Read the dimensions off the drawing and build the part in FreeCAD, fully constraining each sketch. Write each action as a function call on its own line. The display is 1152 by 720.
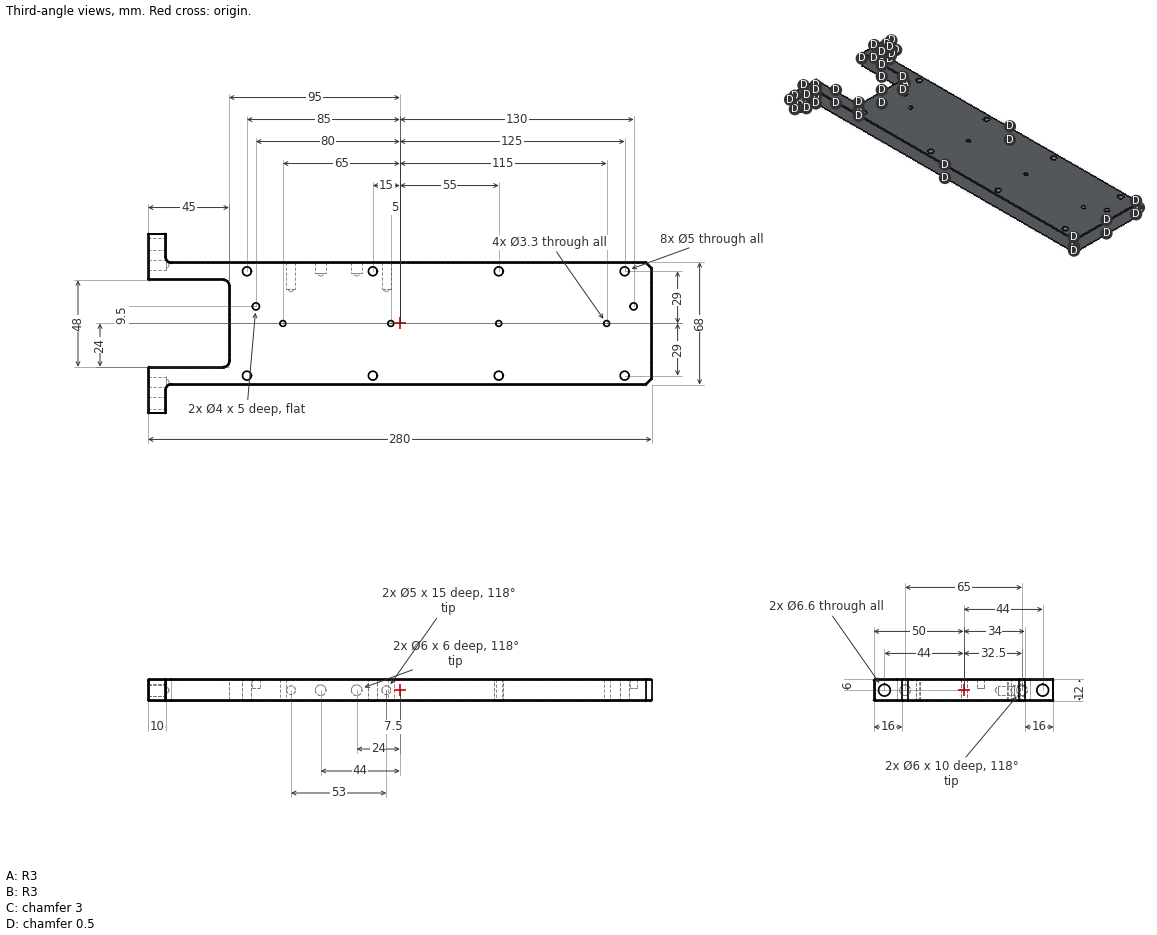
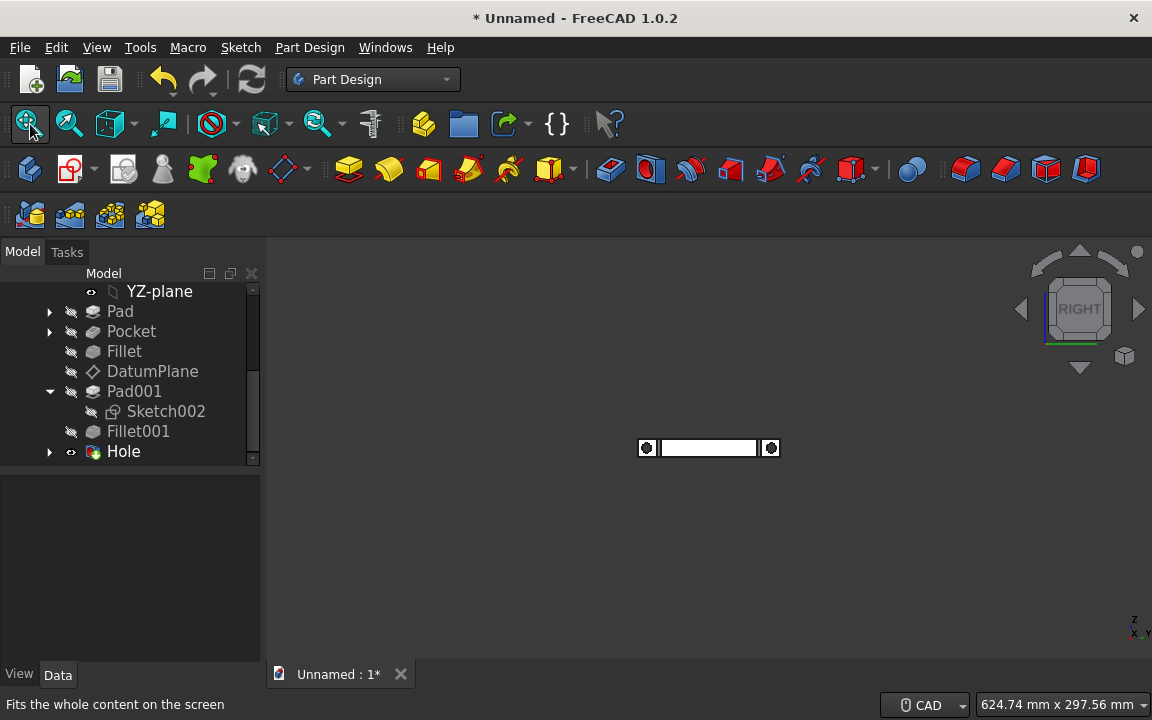
key(6)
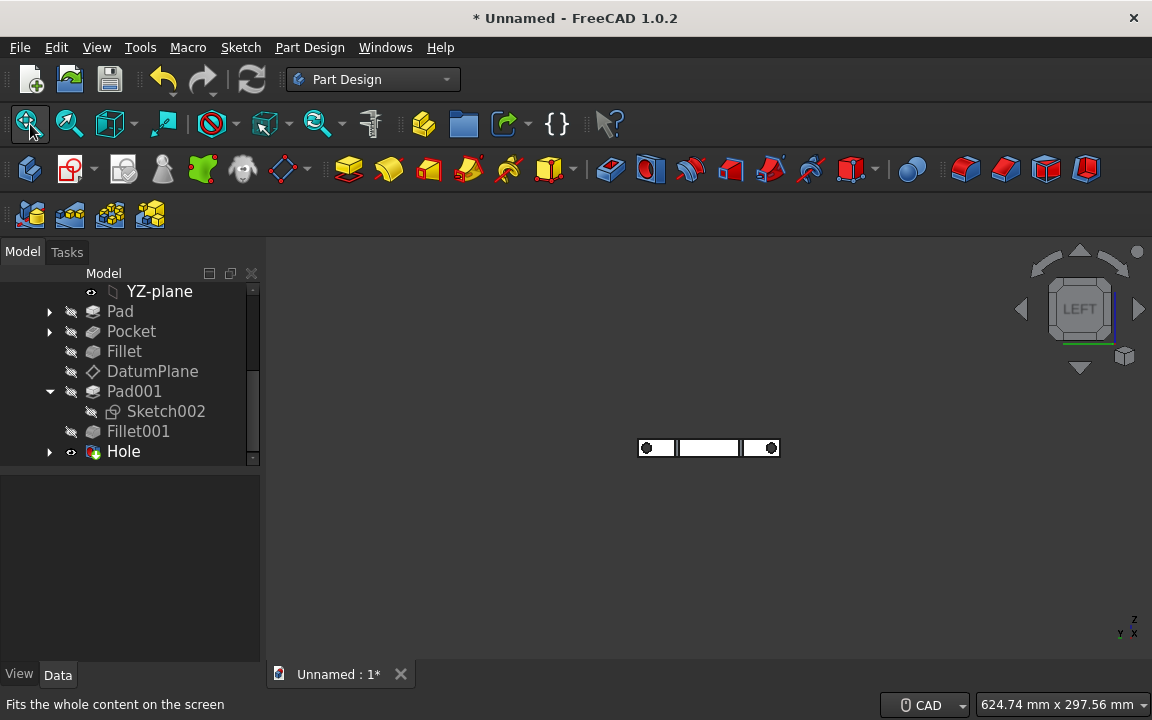
key(v)
key(f)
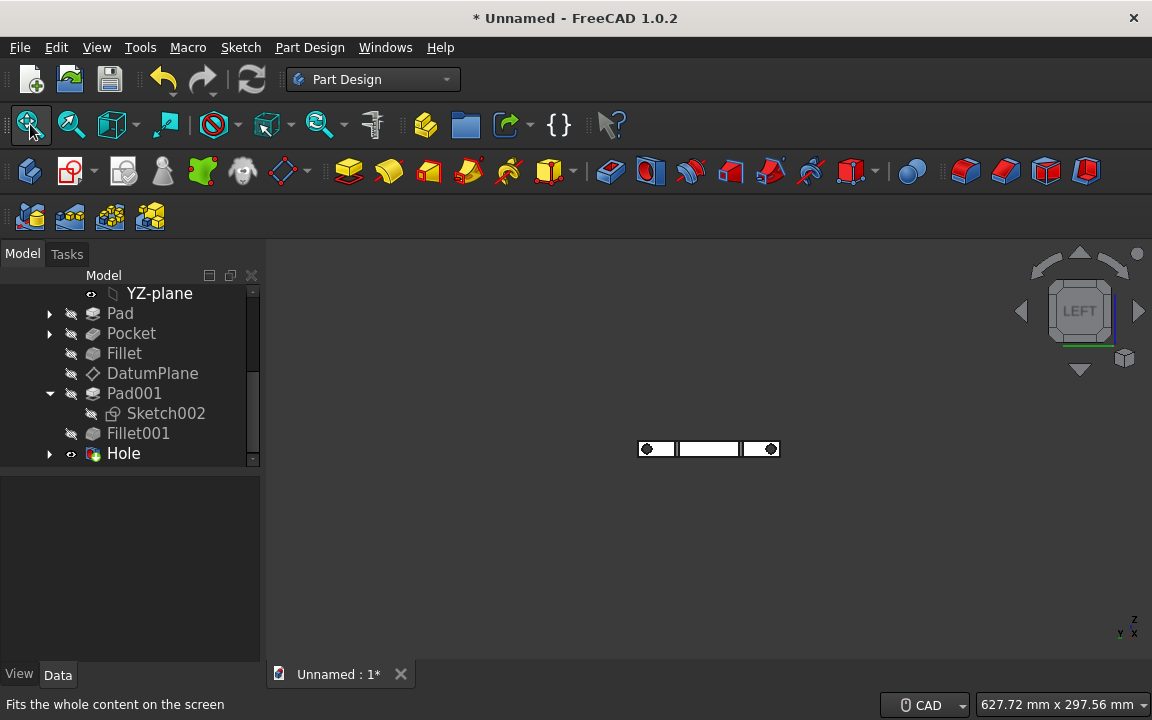
click(662, 448)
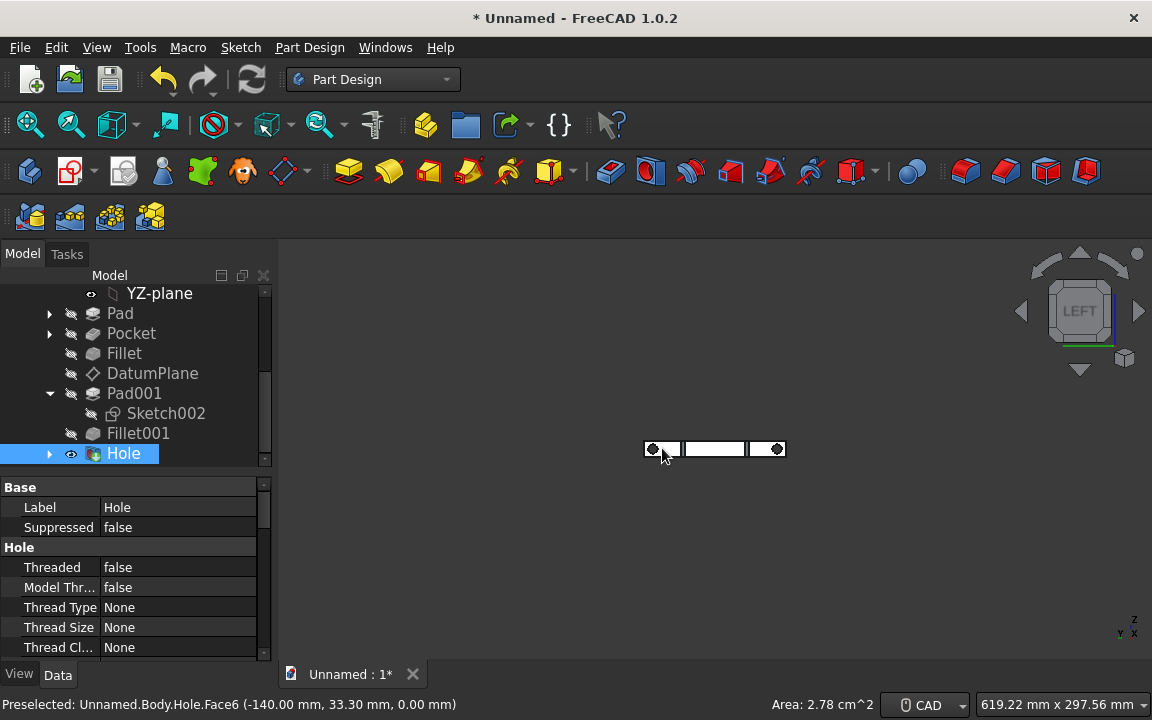
click(70, 172)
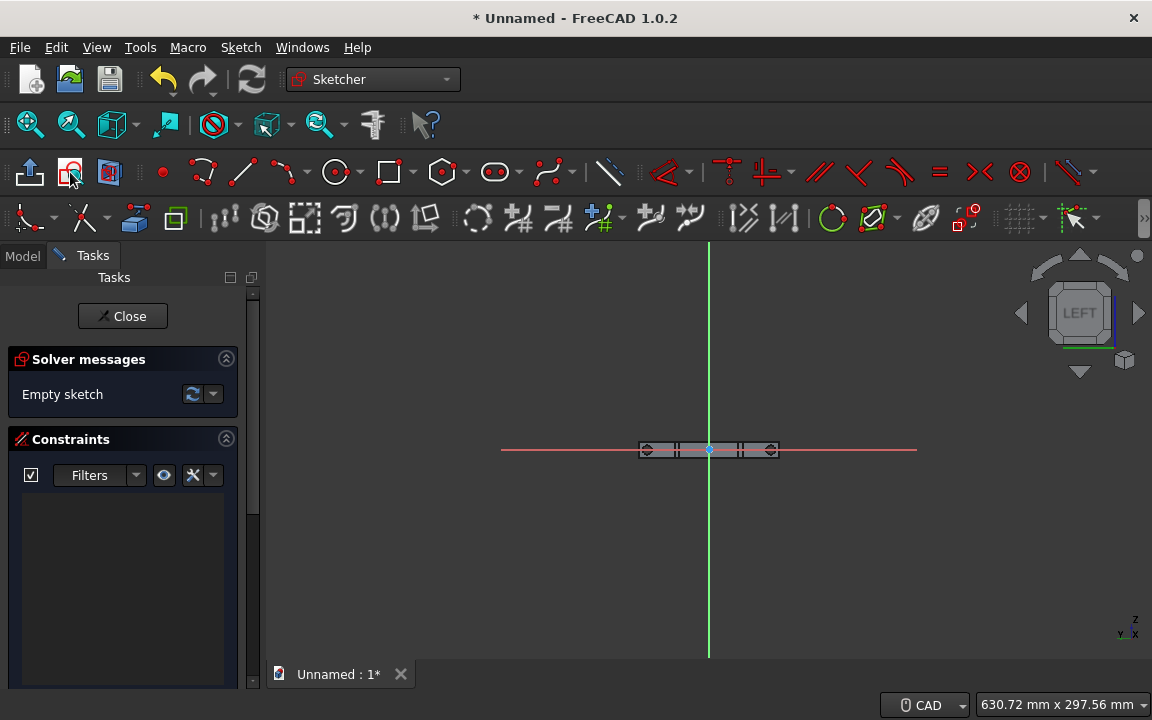
scroll(726, 450, up, 8)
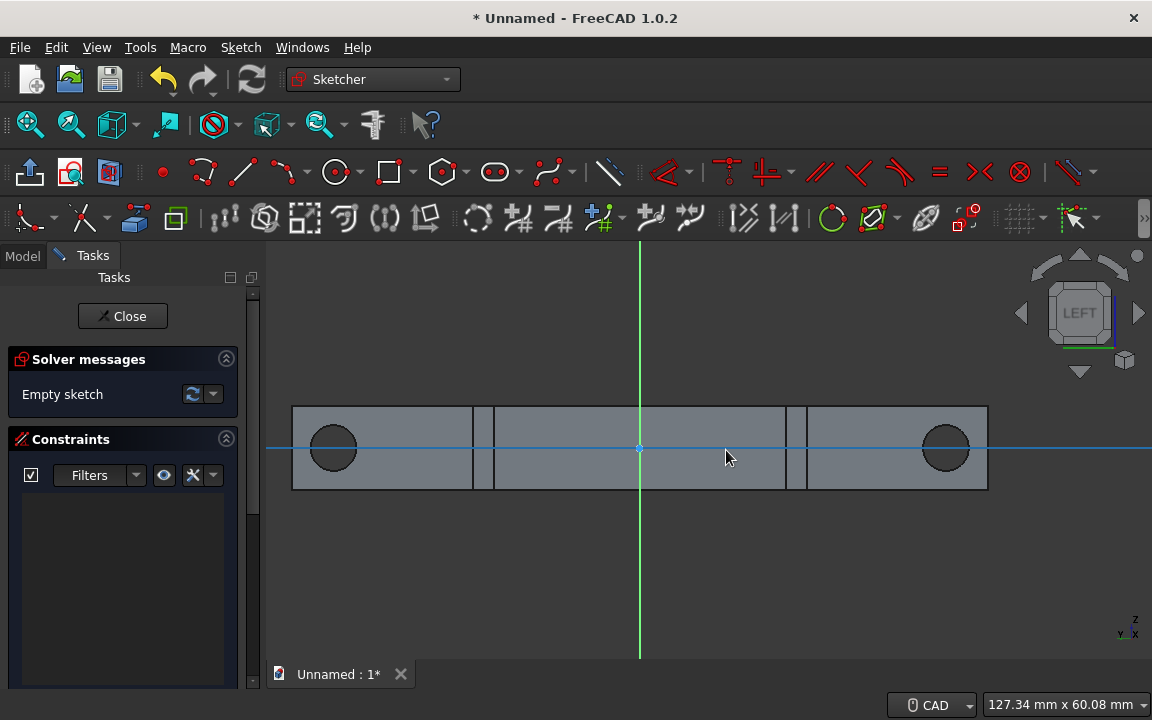
click(336, 172)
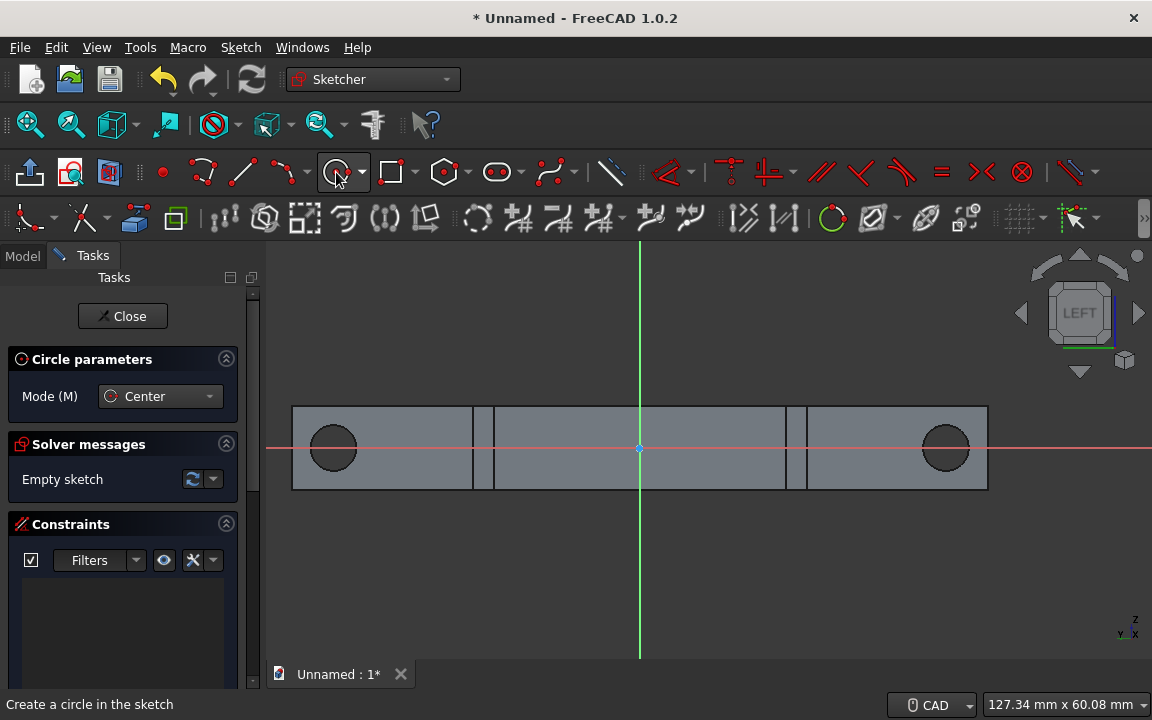
click(414, 448)
move(428, 433)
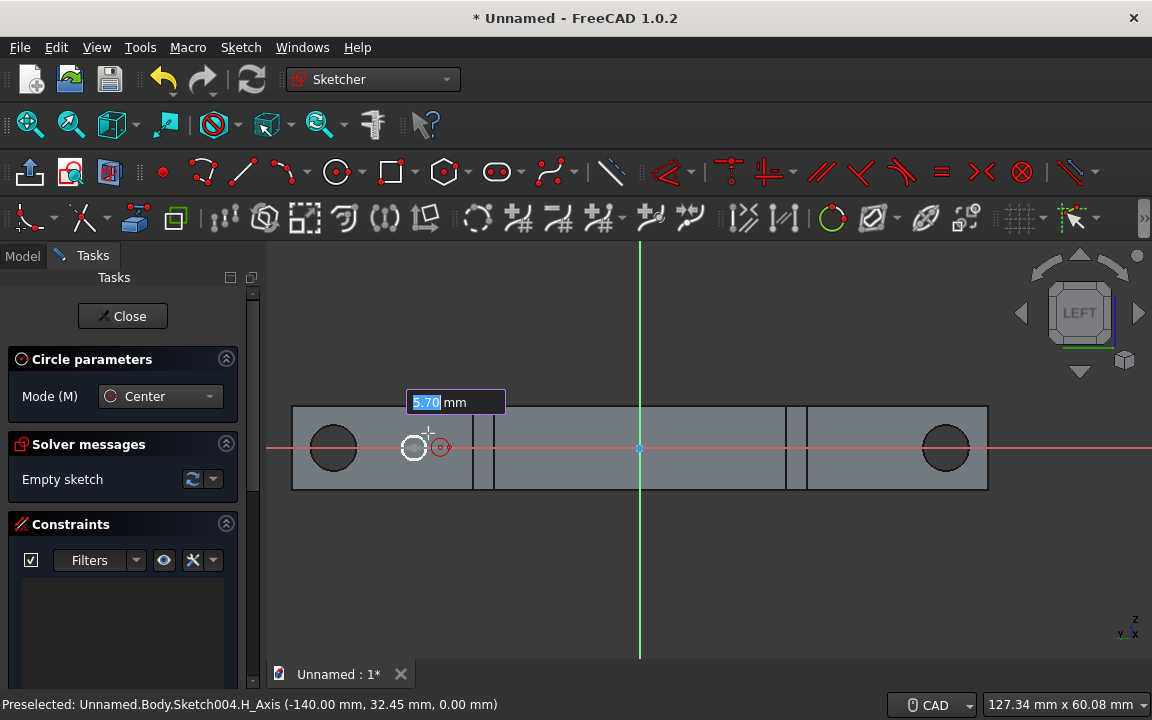
text(6)
key(Return)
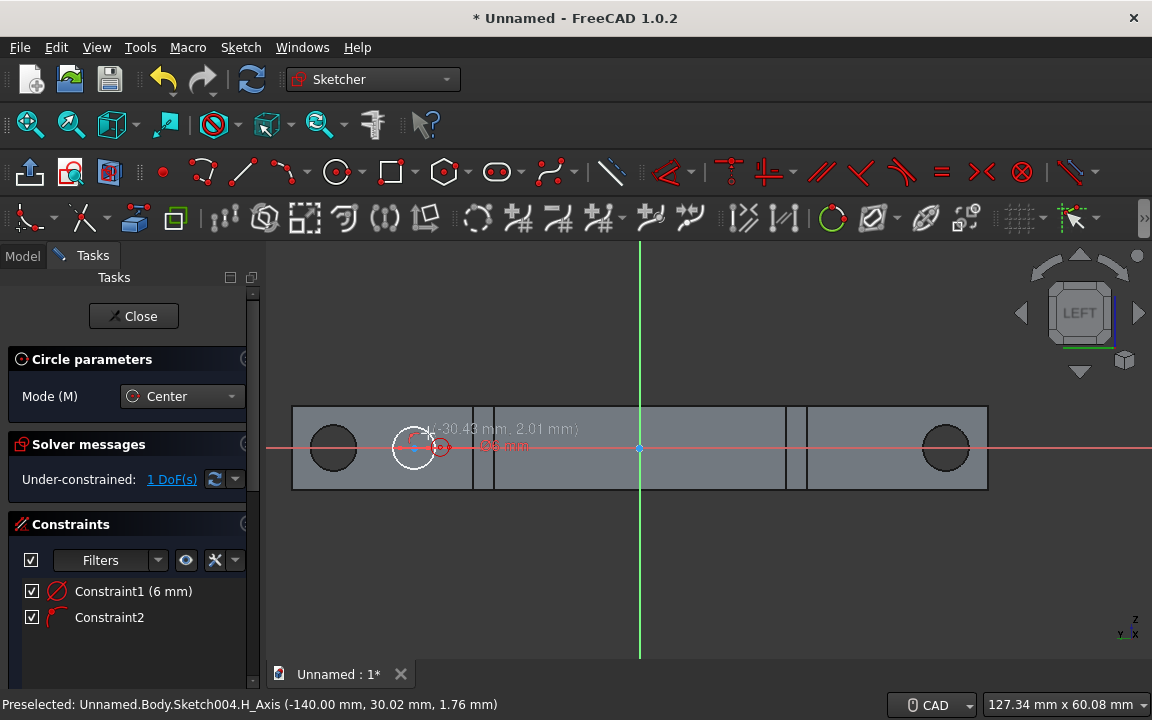
click(866, 448)
move(881, 433)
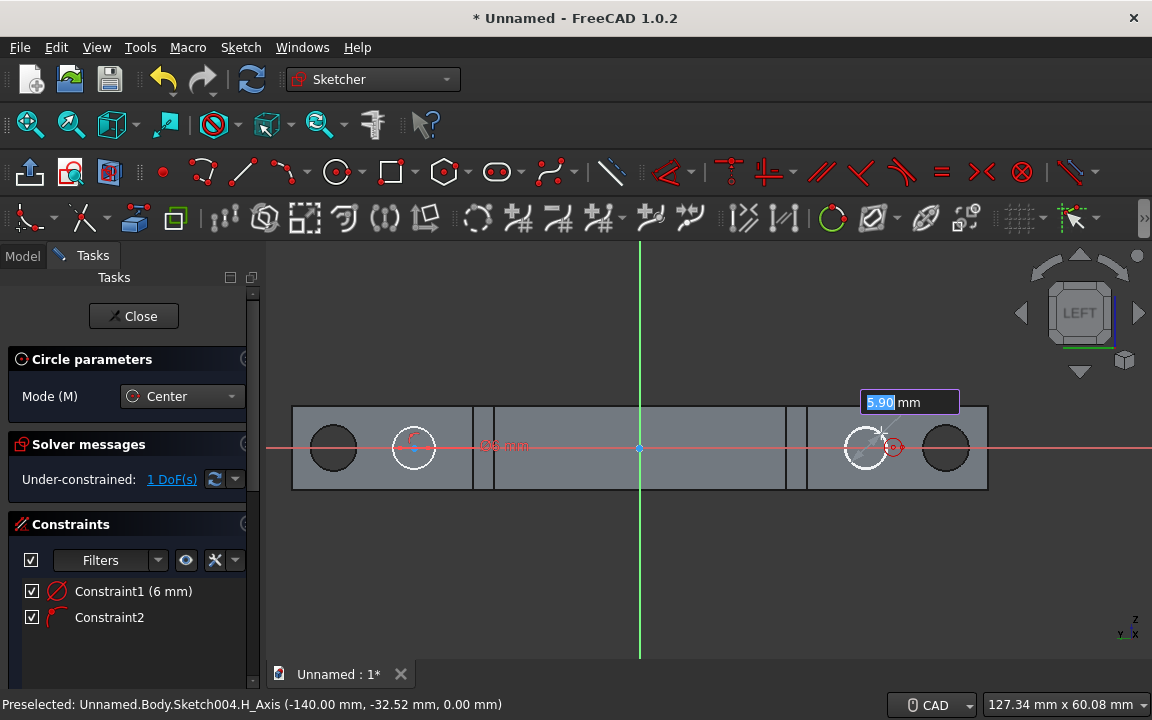
text(6)
key(Return)
key(Escape)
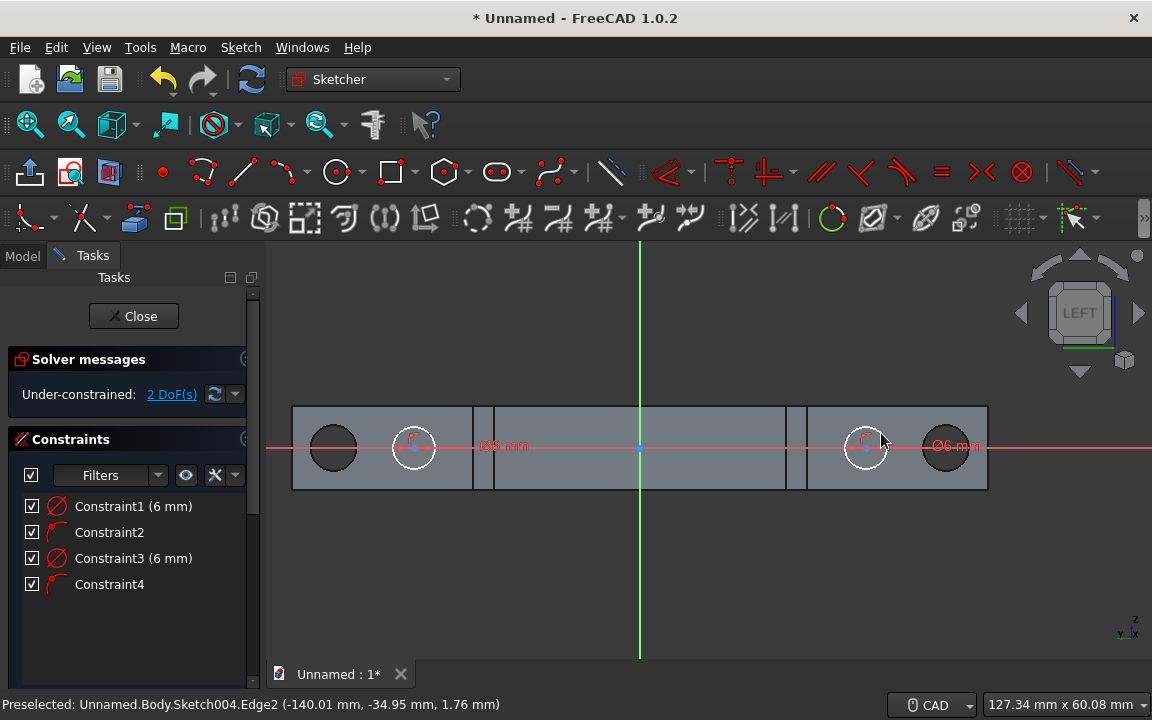
key(d)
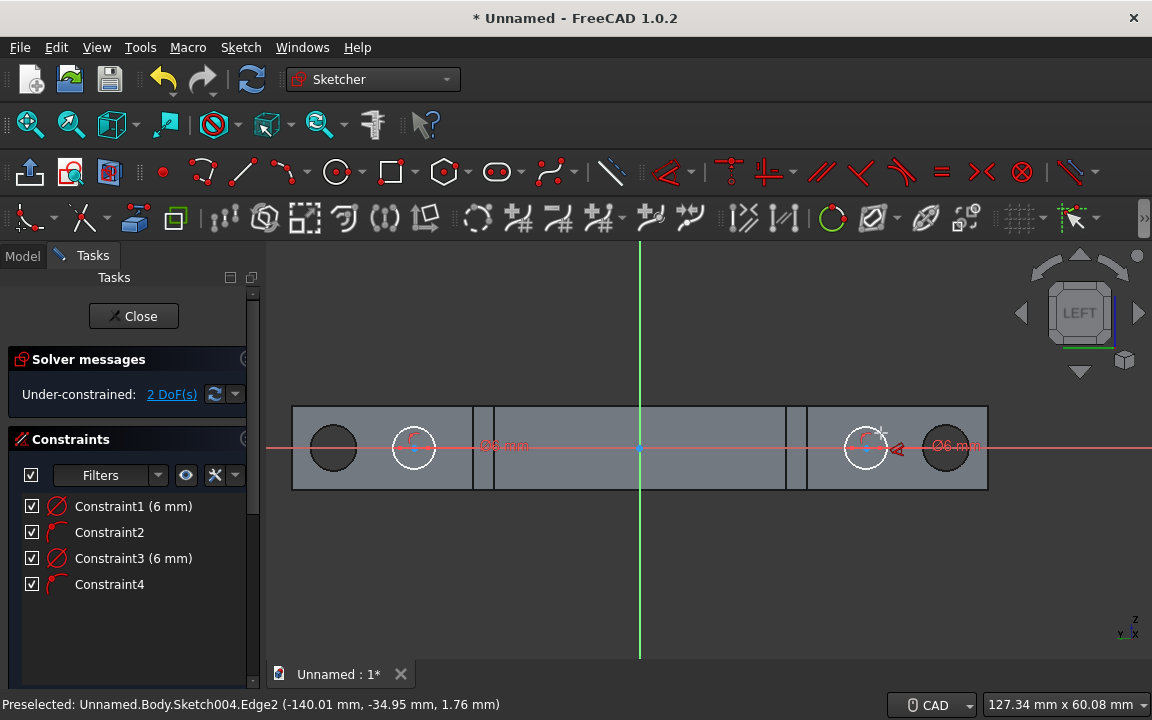
click(414, 448)